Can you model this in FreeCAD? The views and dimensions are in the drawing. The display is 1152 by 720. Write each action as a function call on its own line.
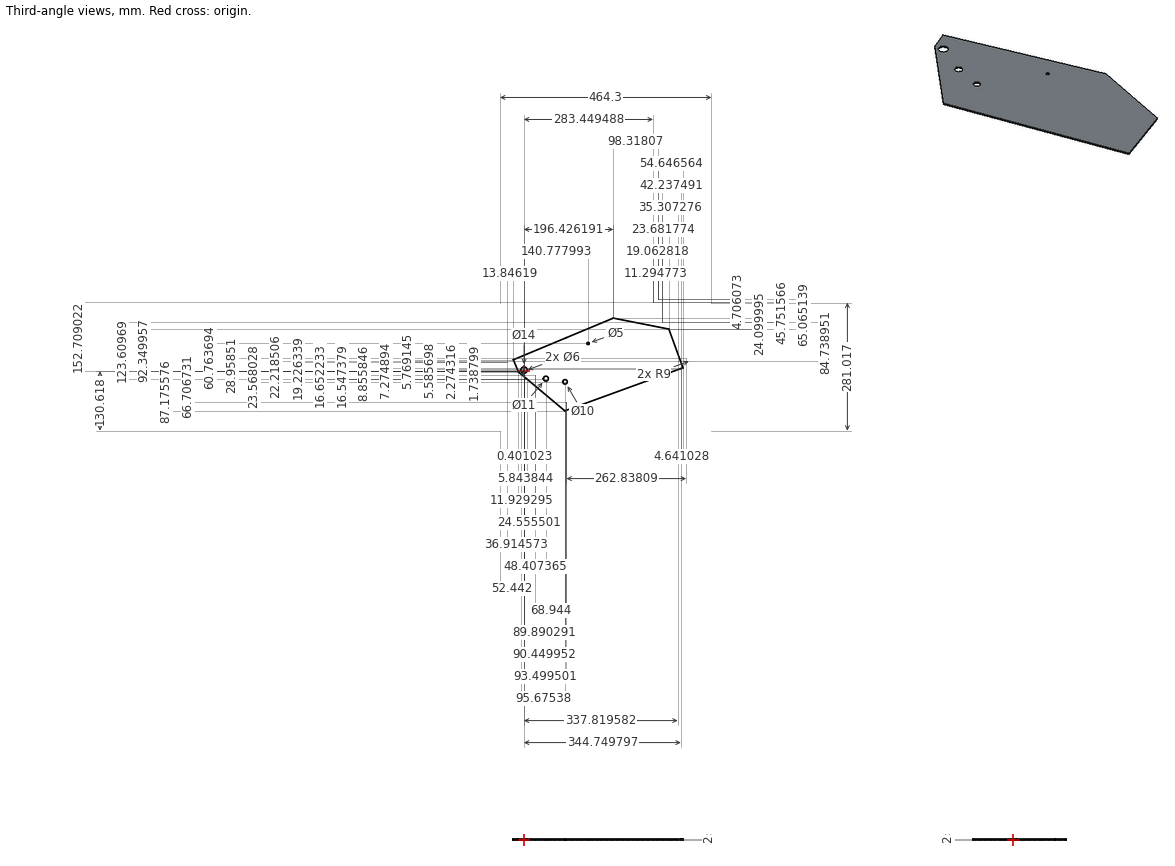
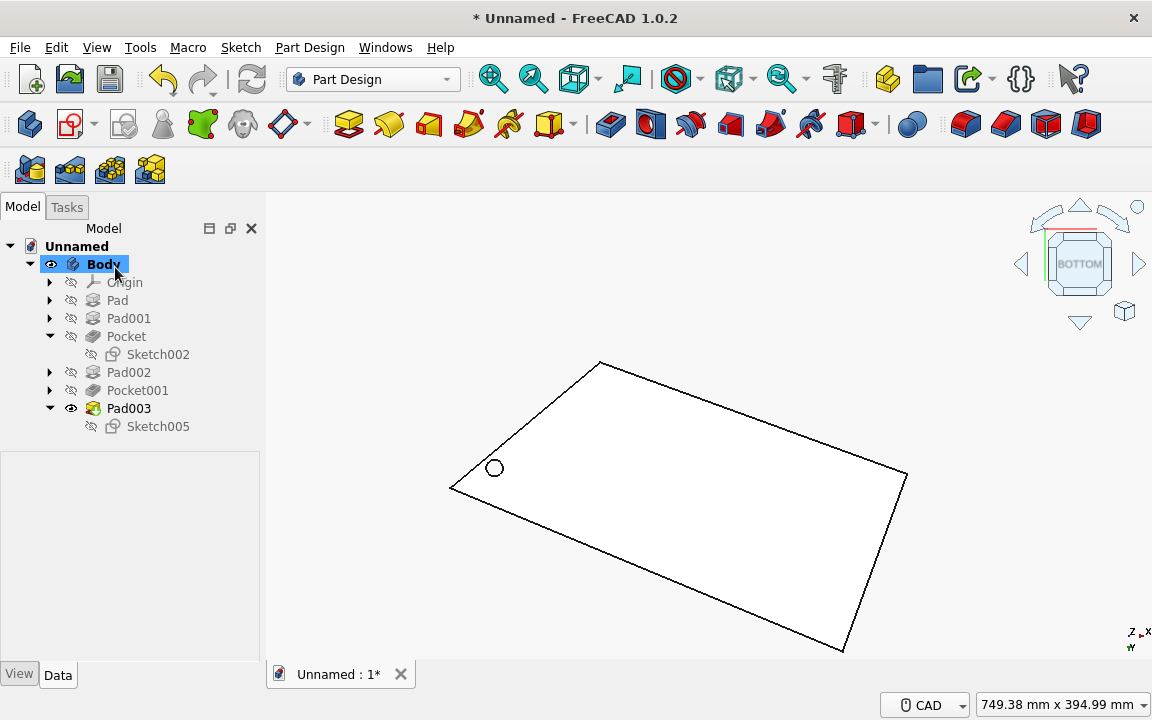
key(0)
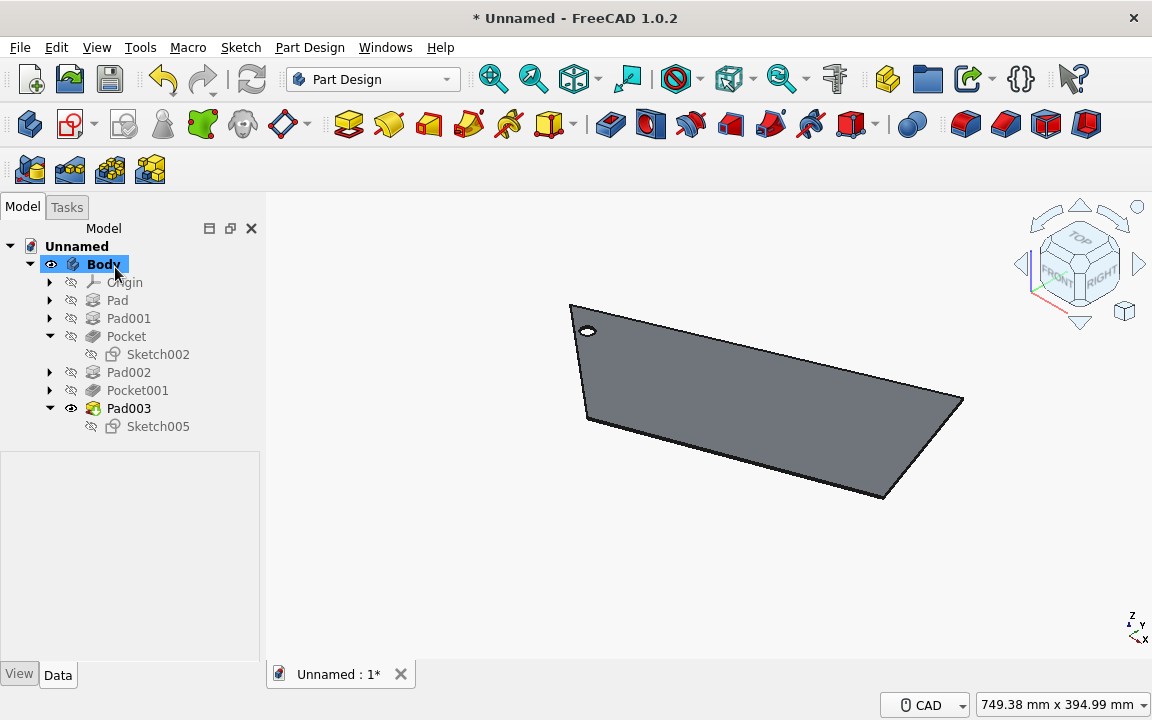
click(791, 416)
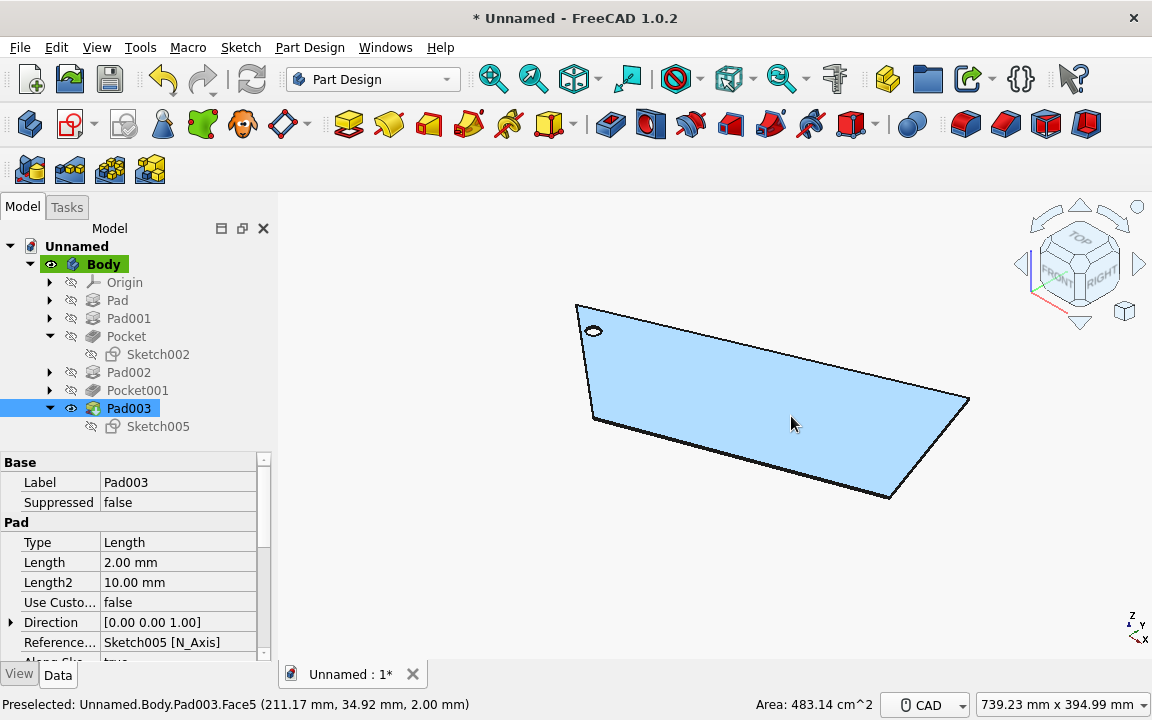
click(70, 124)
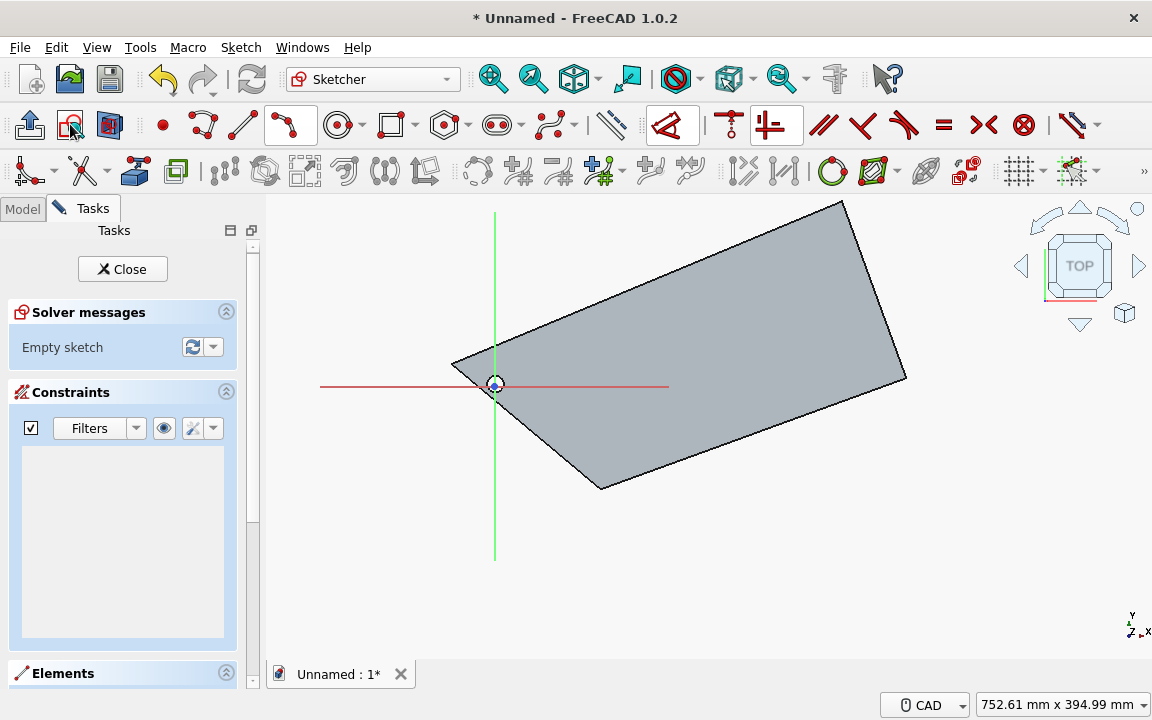
scroll(640, 426, down, 5)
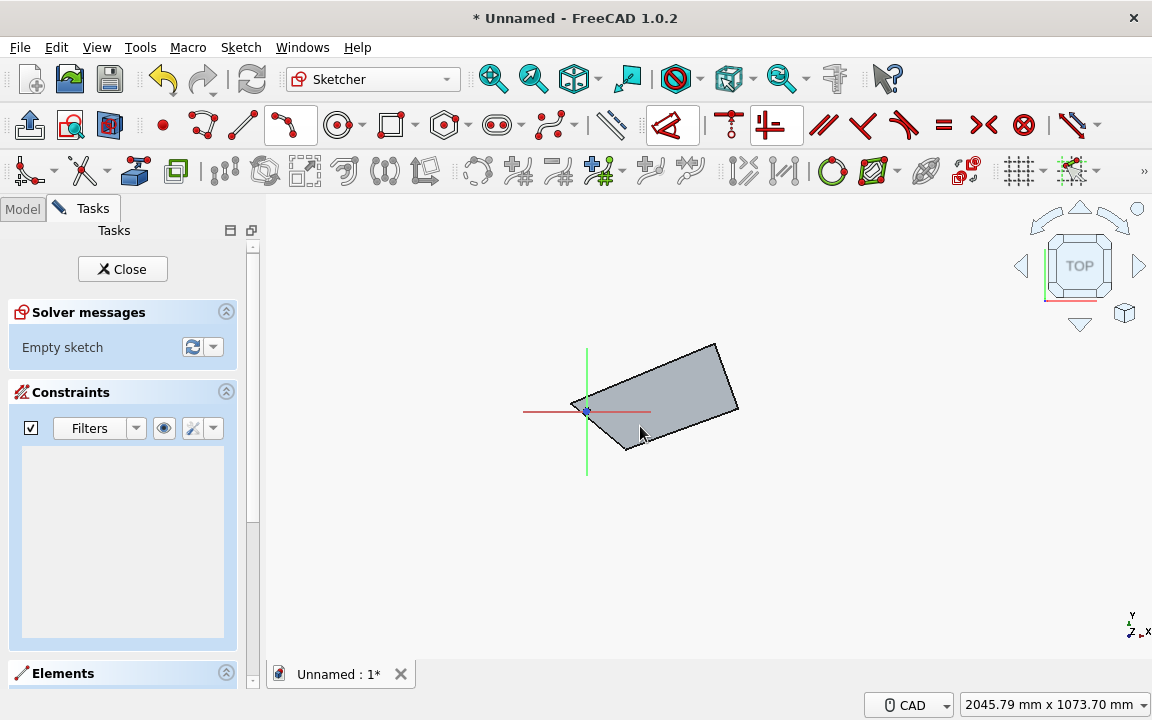
scroll(706, 349, up, 11)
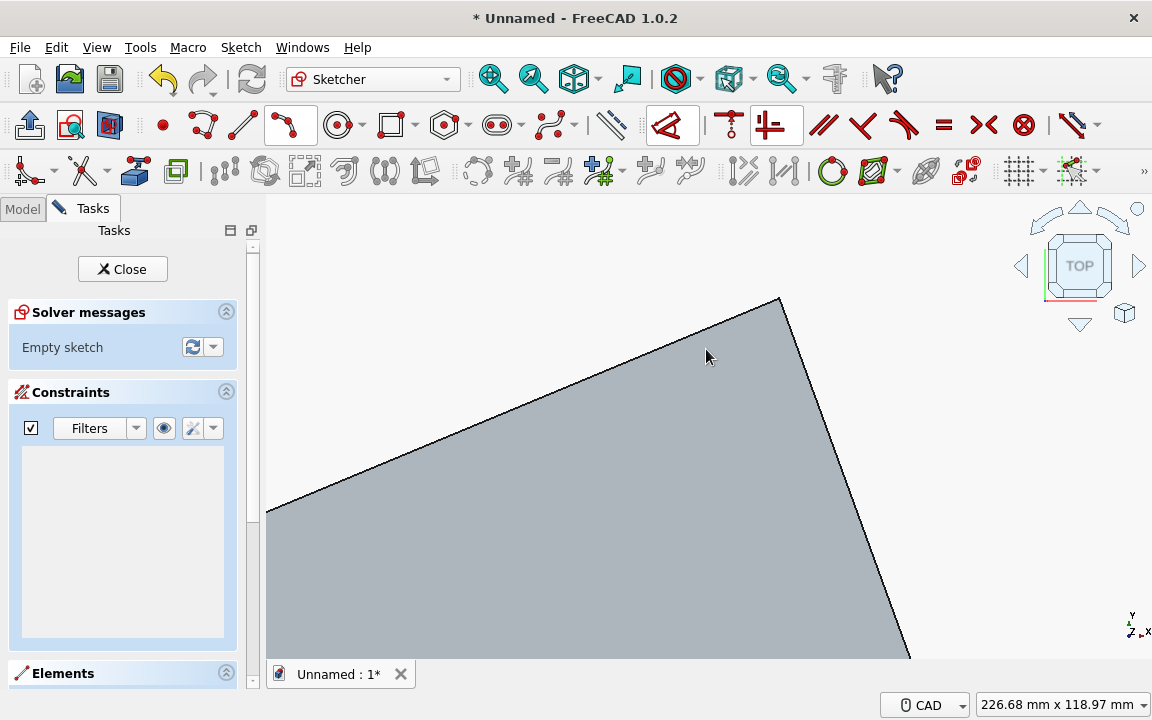
click(204, 126)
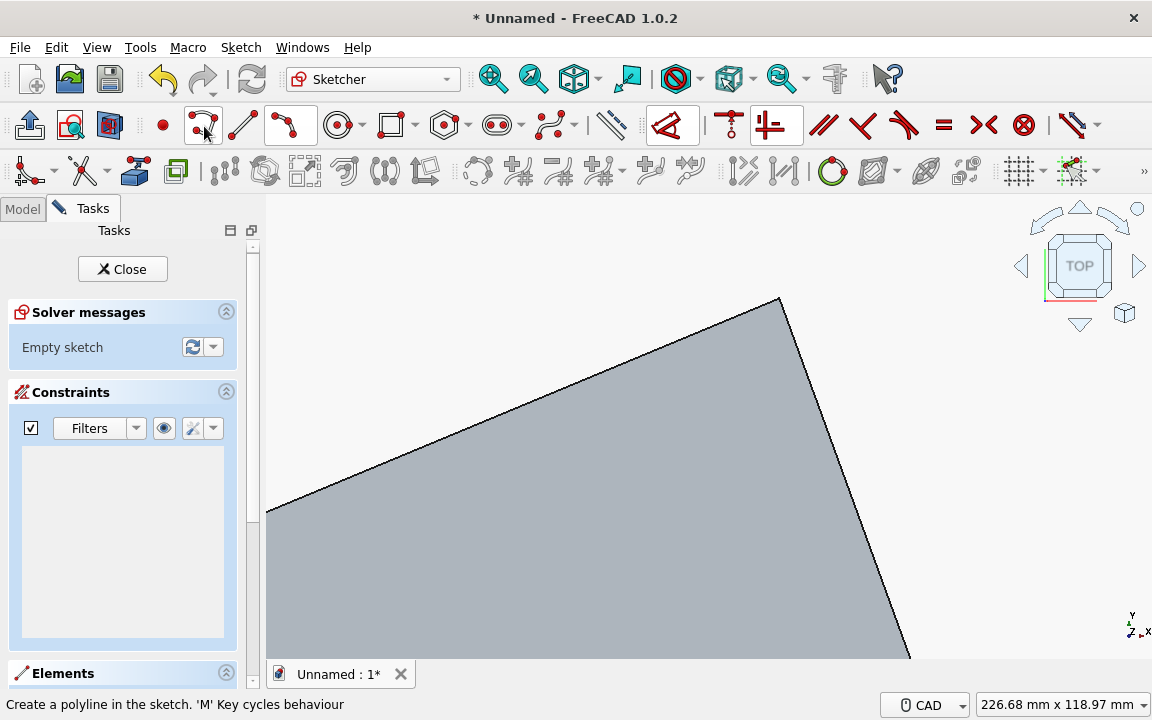
click(395, 459)
click(872, 553)
click(779, 298)
click(395, 460)
key(Escape)
key(Escape)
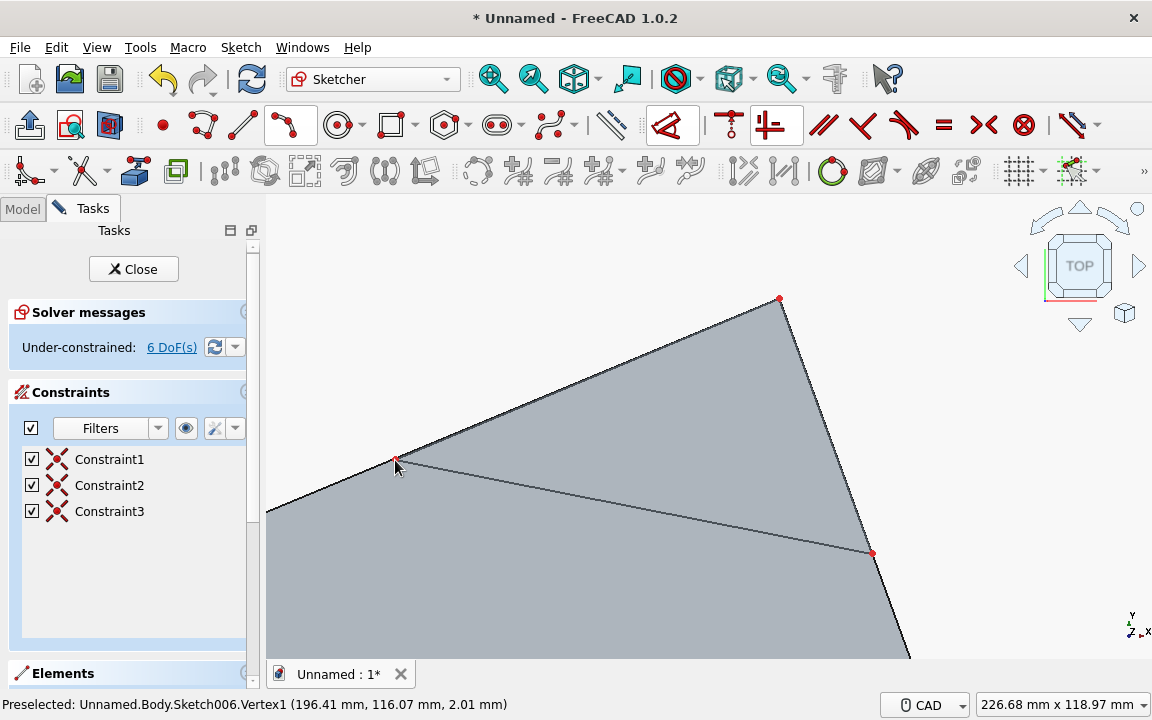
click(664, 347)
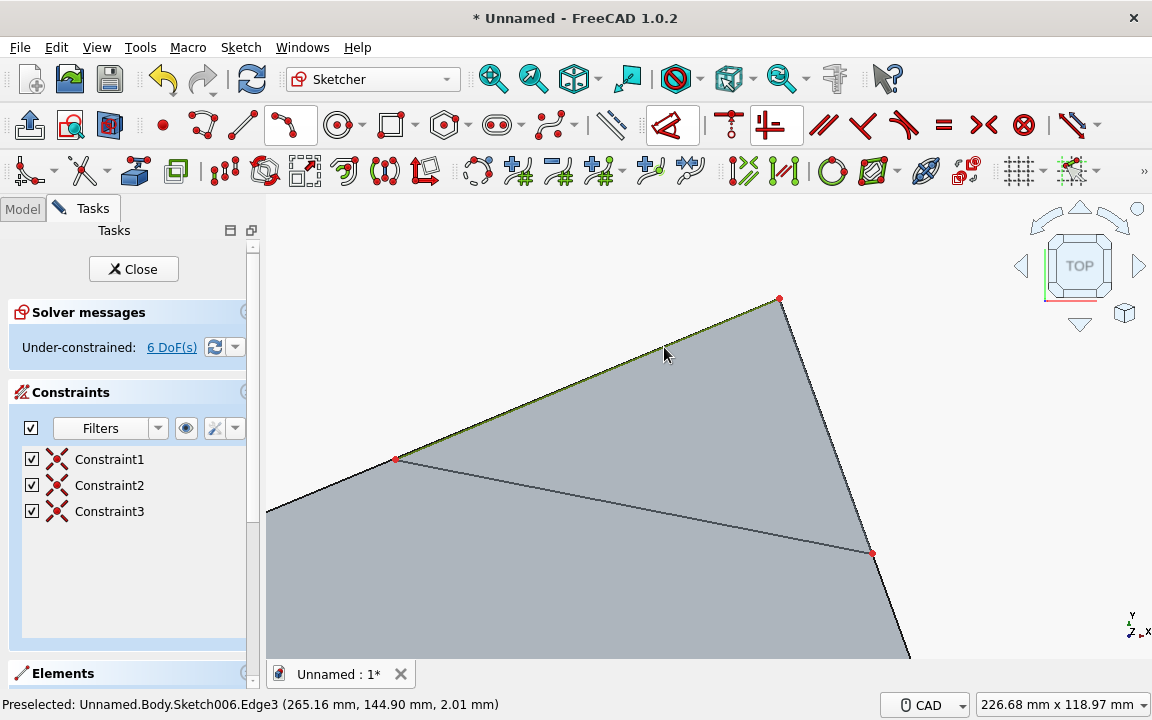
key(l)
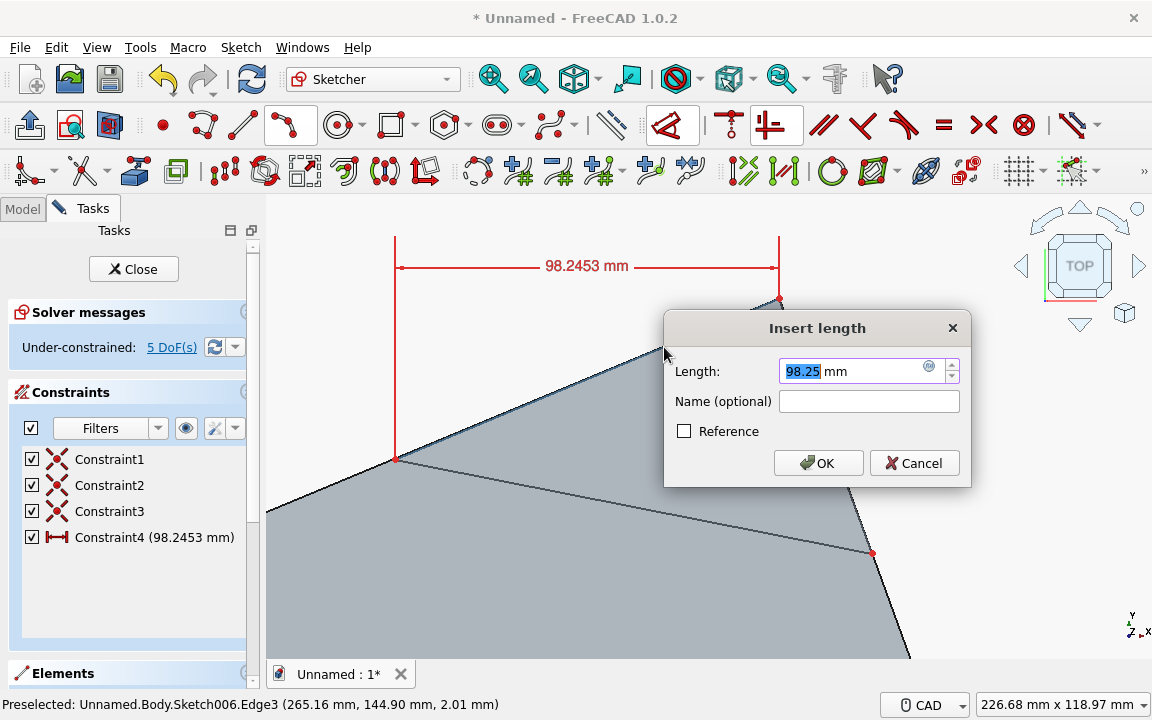
text(98.31807)
key(Return)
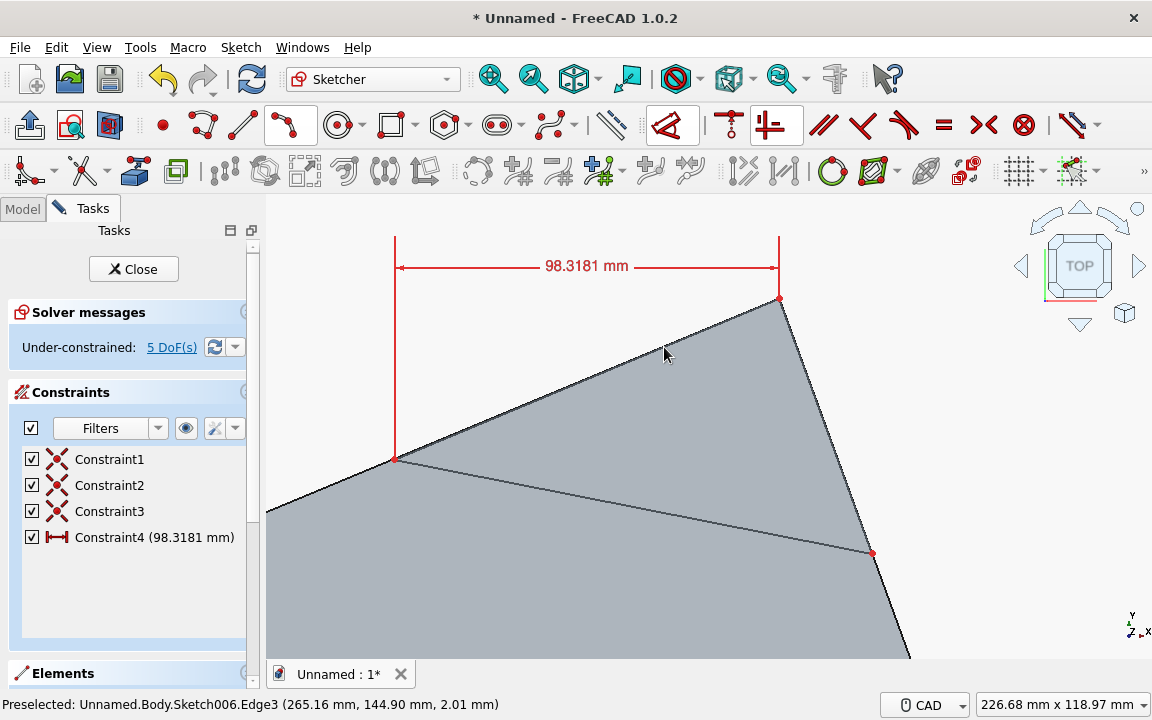
click(872, 554)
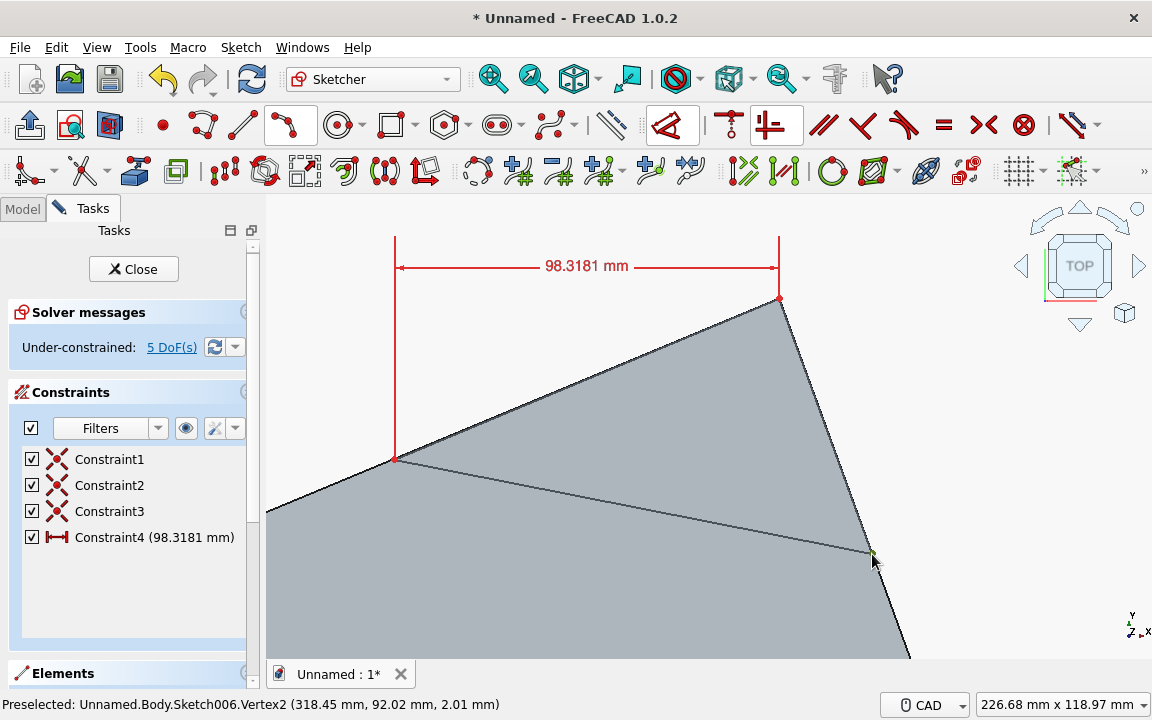
key(i)